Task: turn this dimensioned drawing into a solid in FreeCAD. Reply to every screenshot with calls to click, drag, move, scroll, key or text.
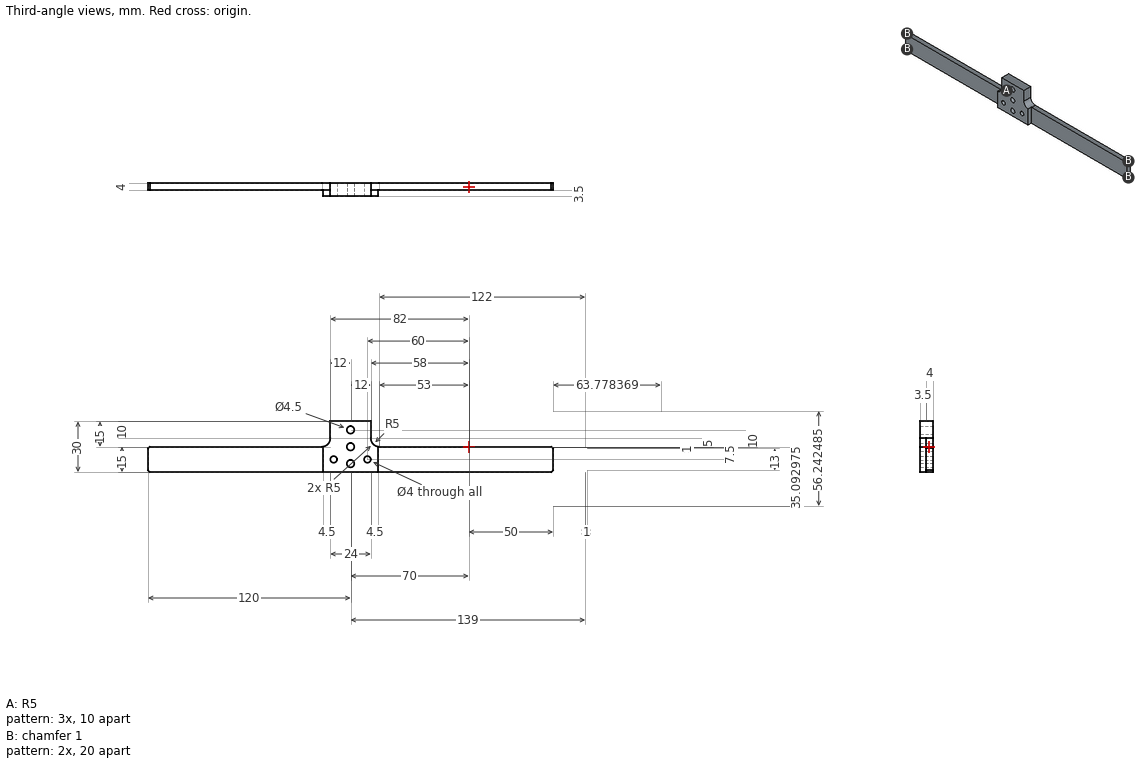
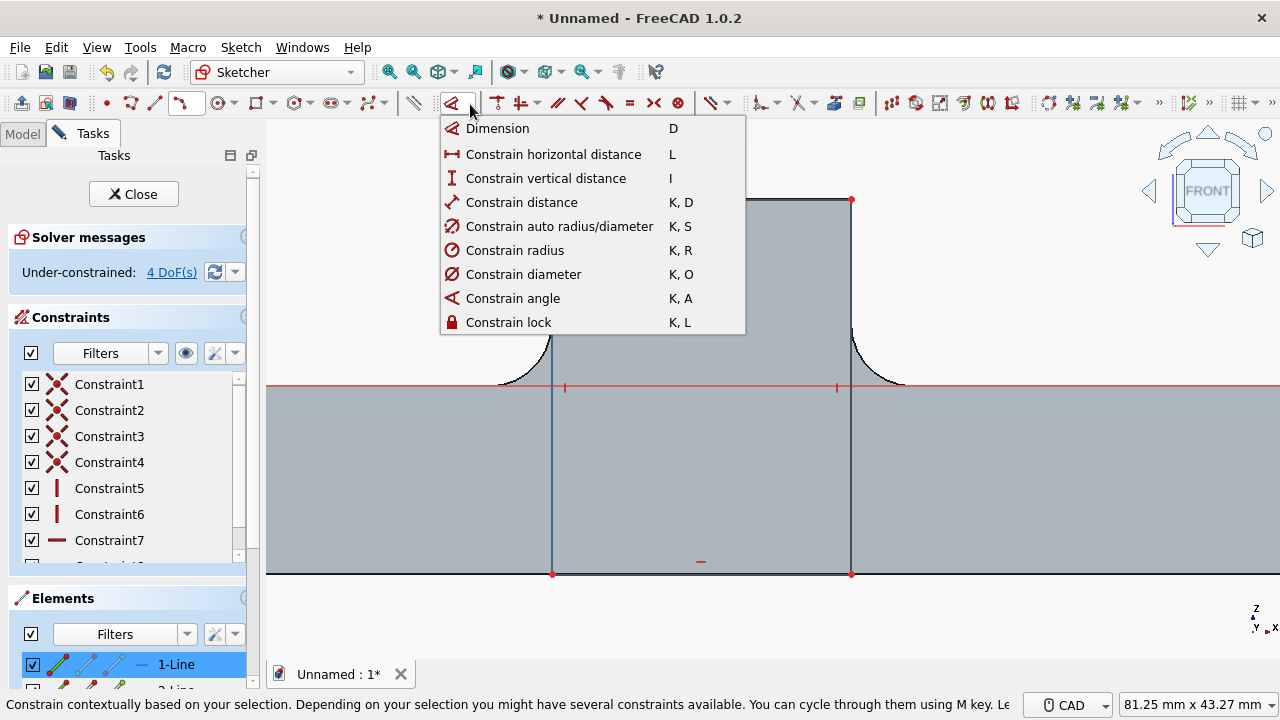
click(593, 178)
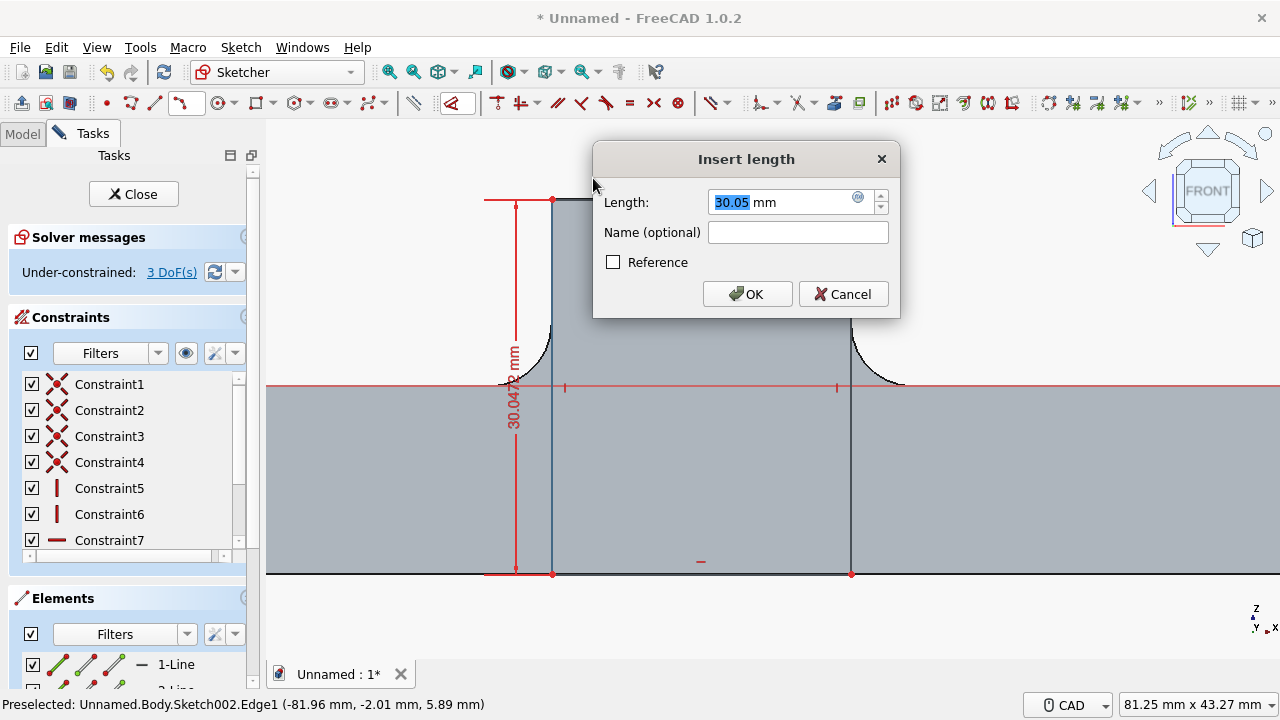
text(30)
key(Return)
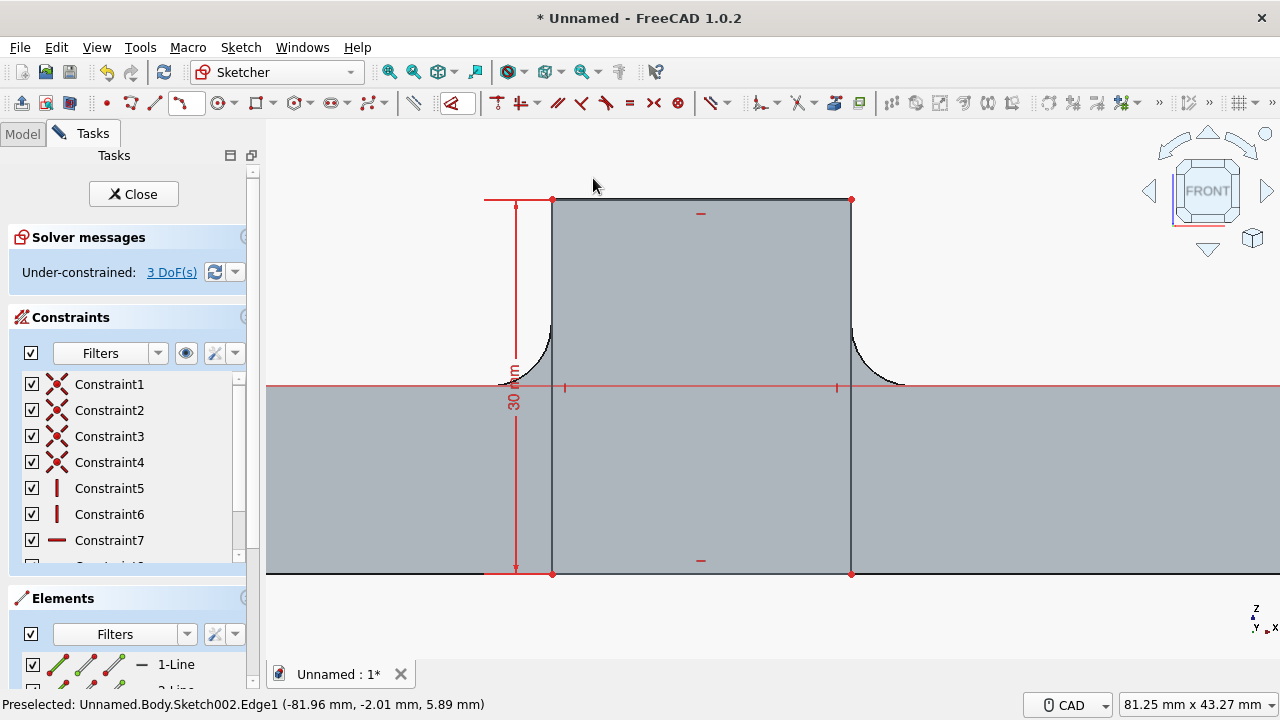
click(642, 574)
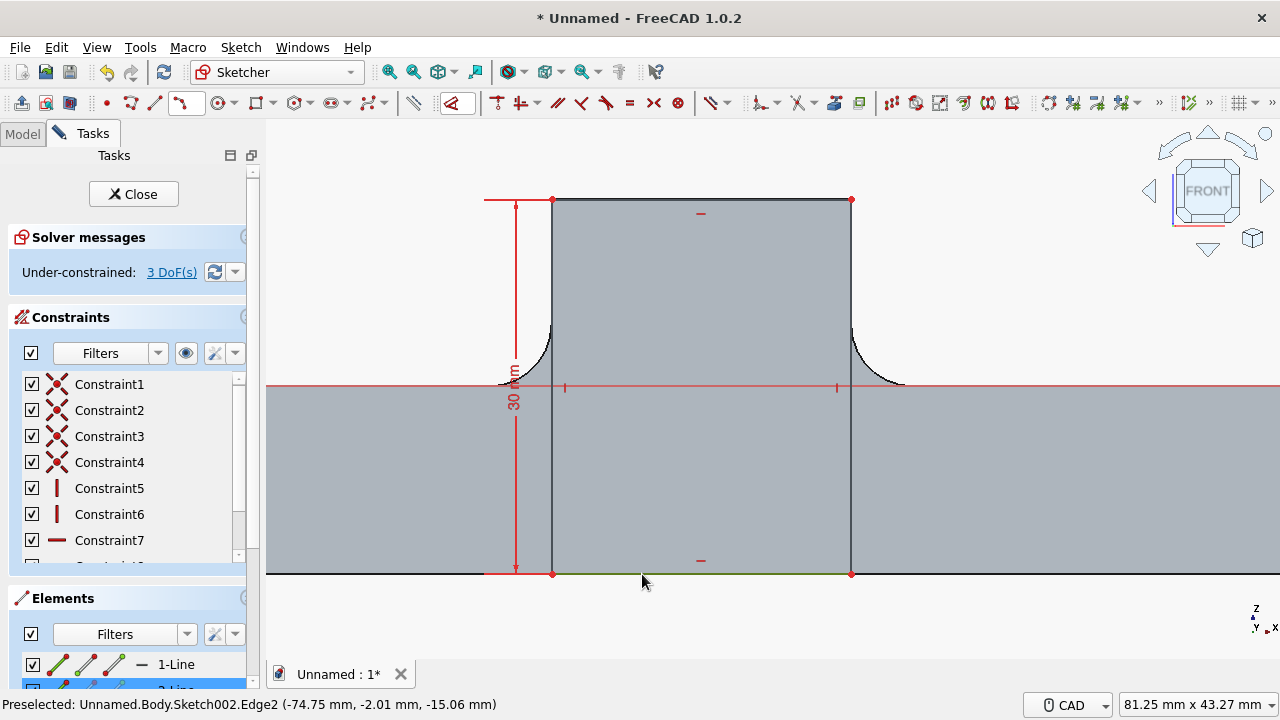
click(470, 104)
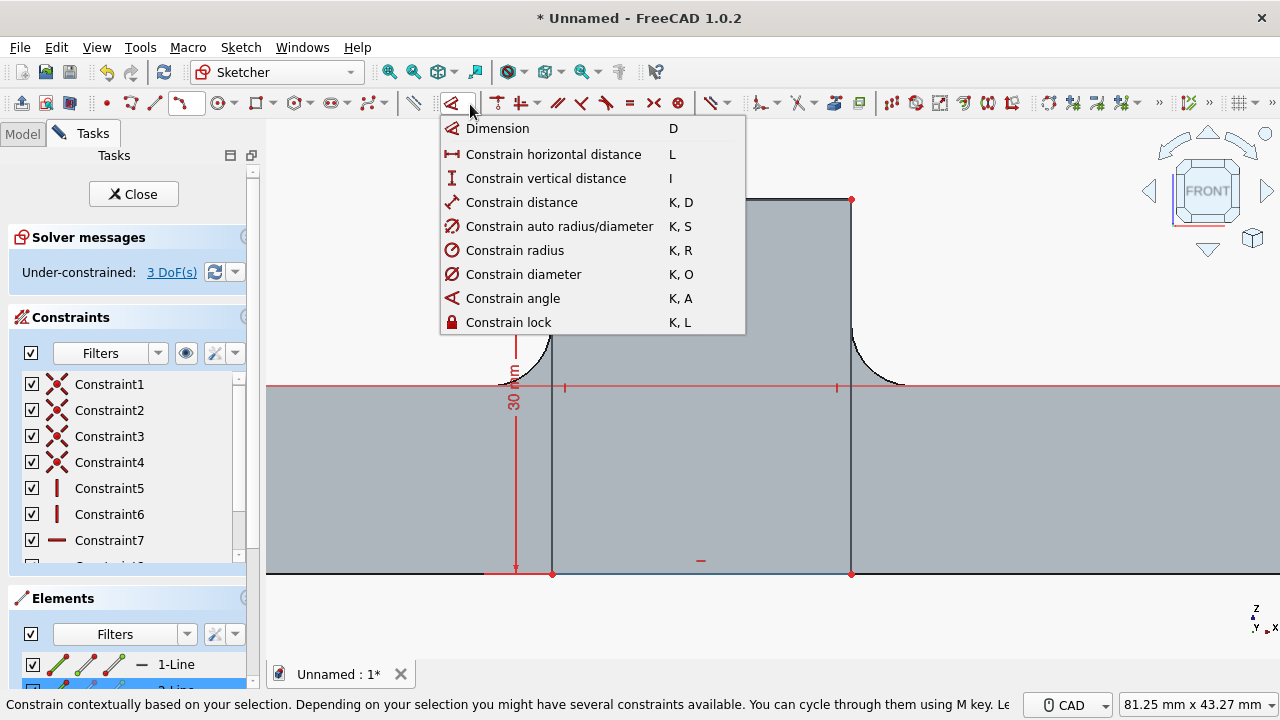
click(593, 154)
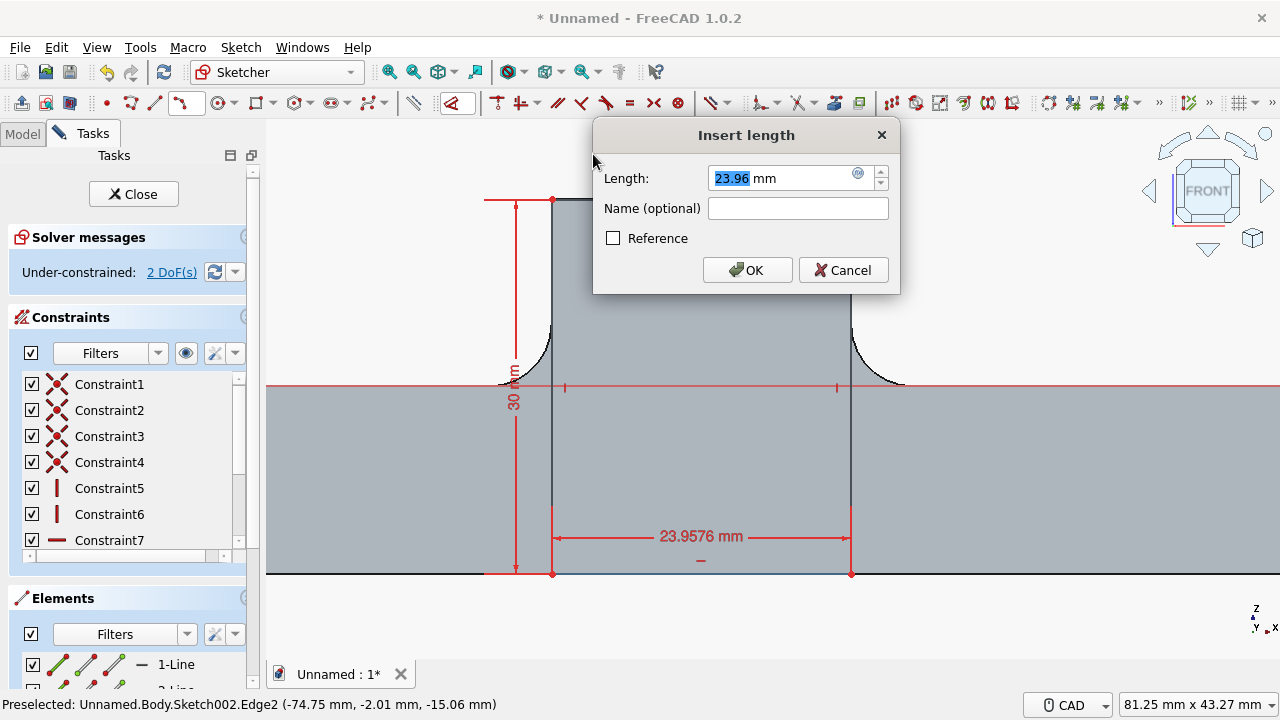
text(24)
key(Return)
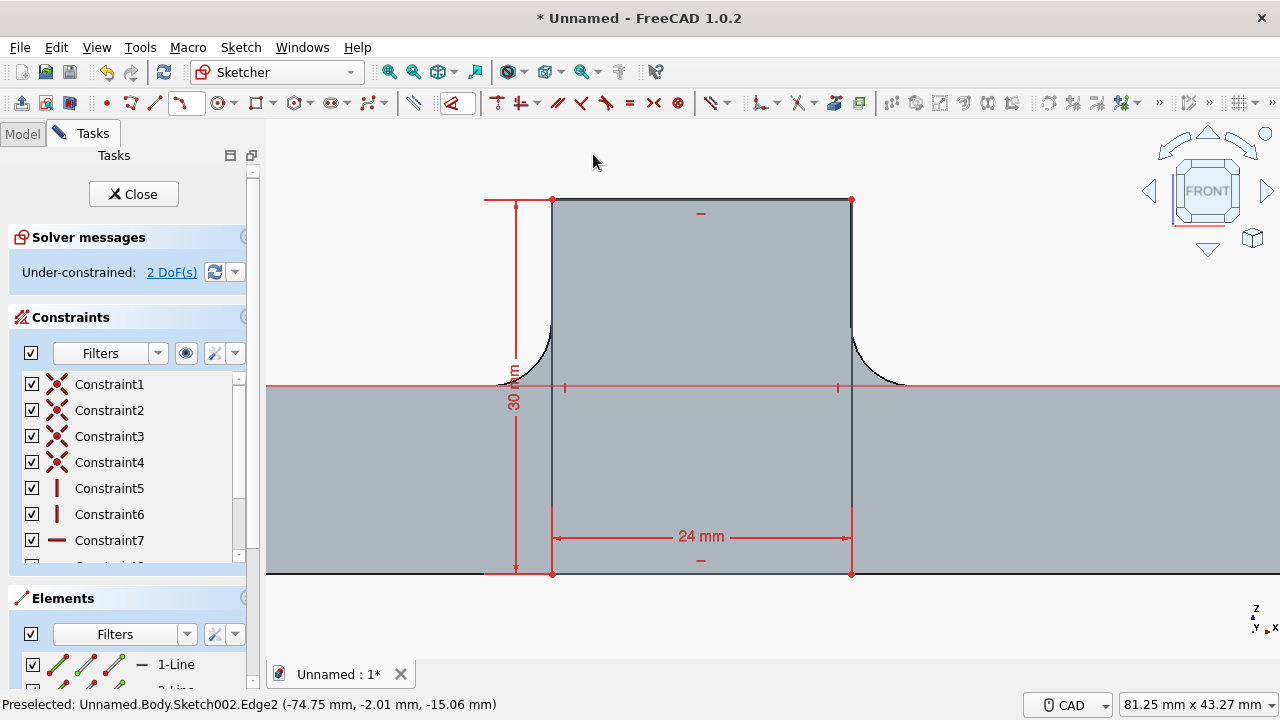
click(552, 200)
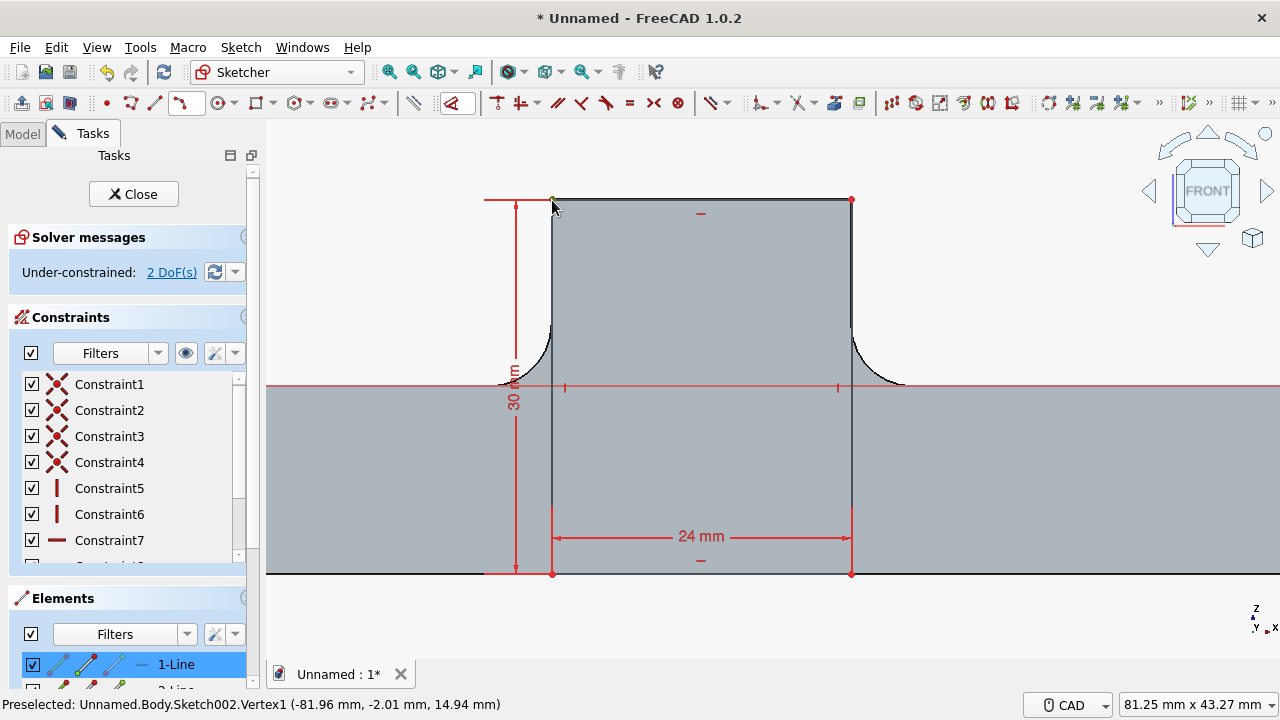
key(l)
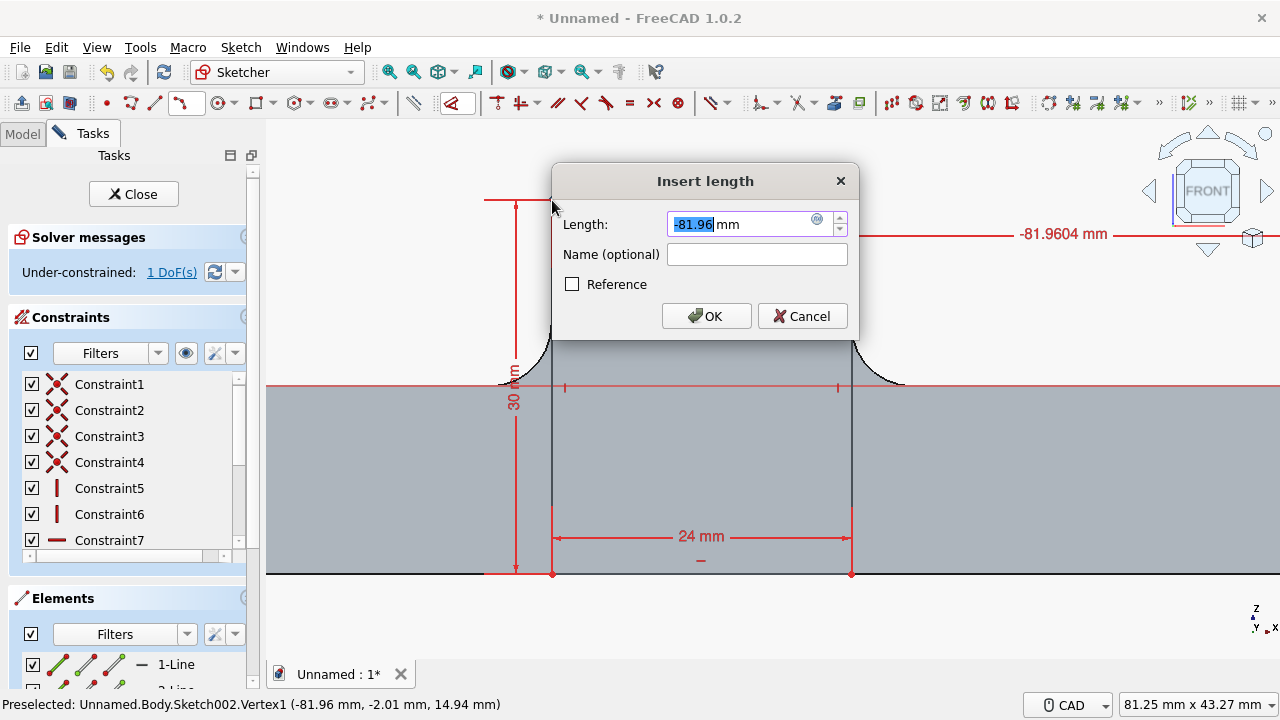
text(-82)
key(Return)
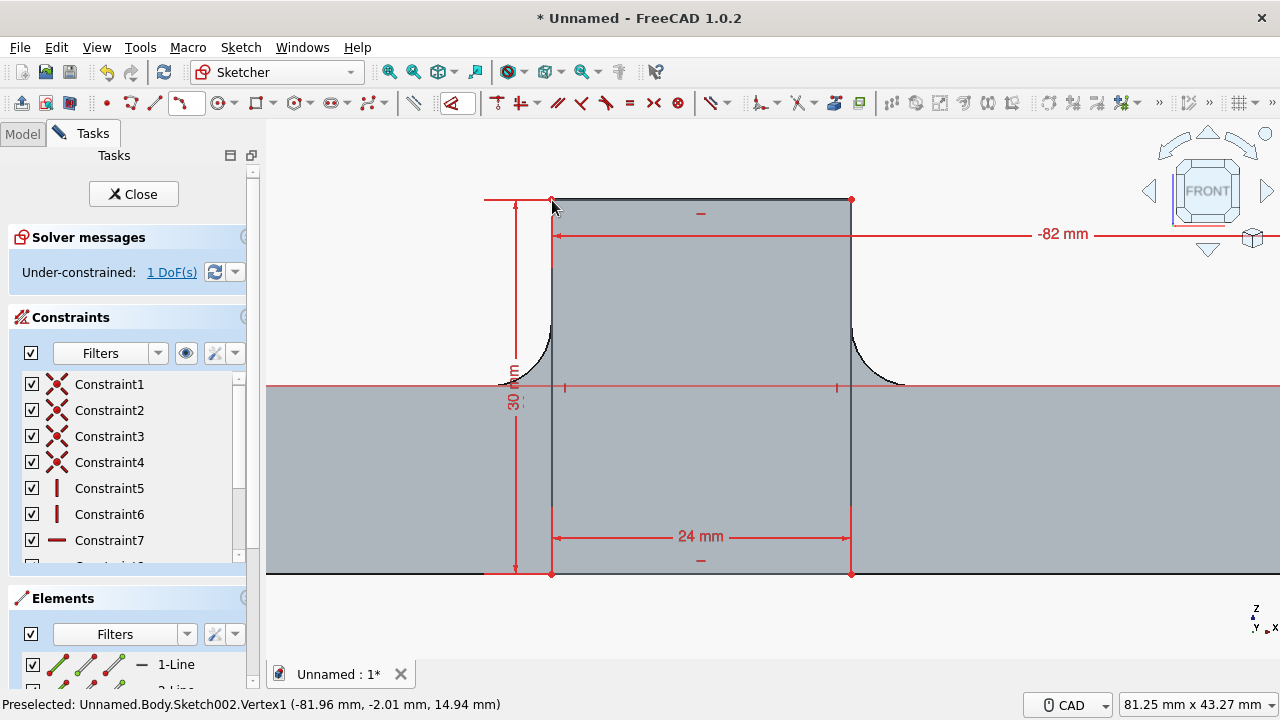
click(552, 200)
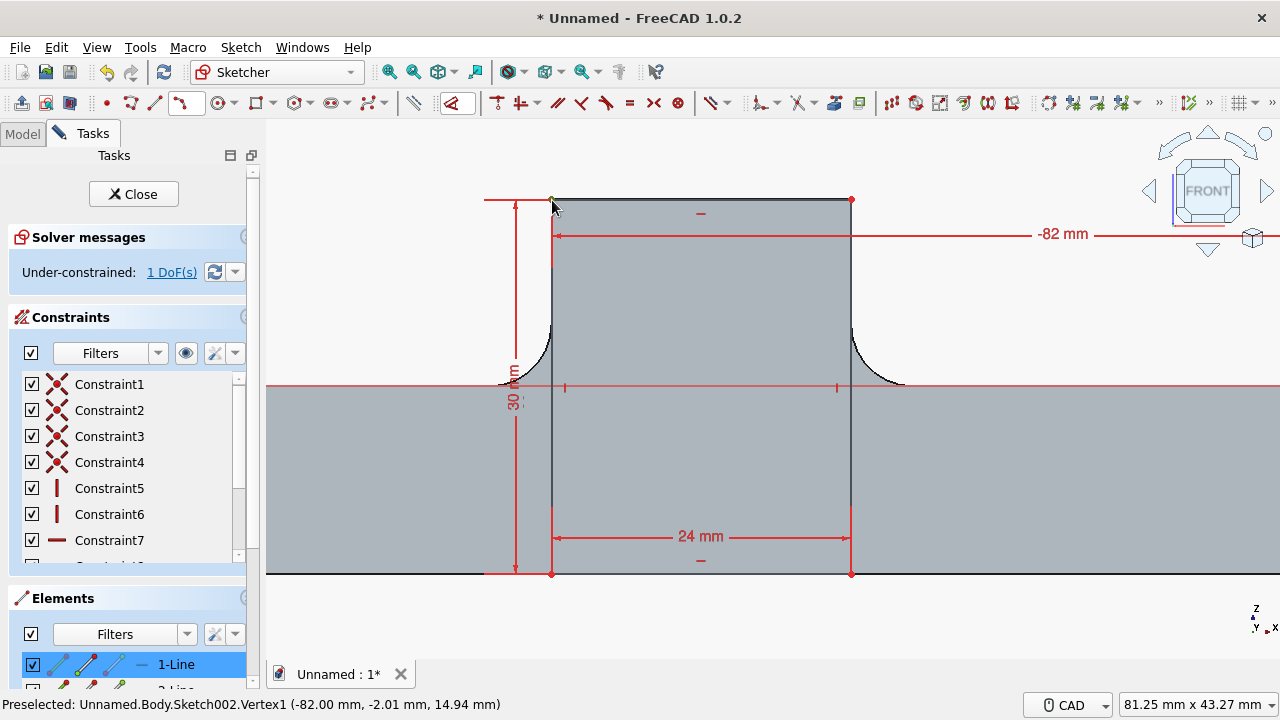
key(i)